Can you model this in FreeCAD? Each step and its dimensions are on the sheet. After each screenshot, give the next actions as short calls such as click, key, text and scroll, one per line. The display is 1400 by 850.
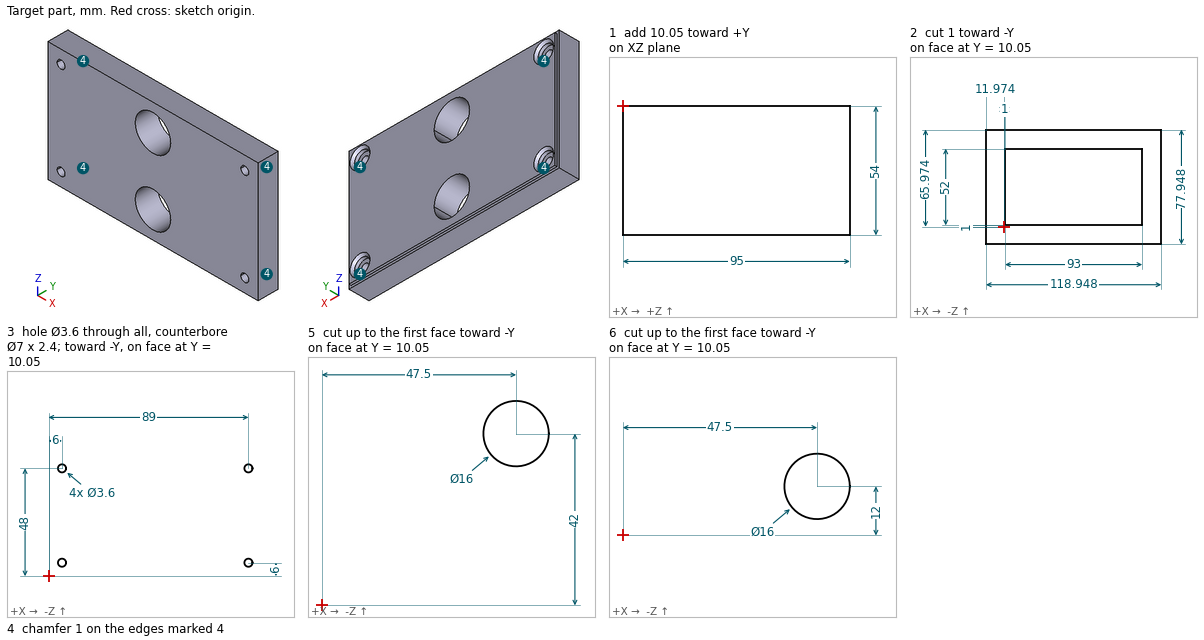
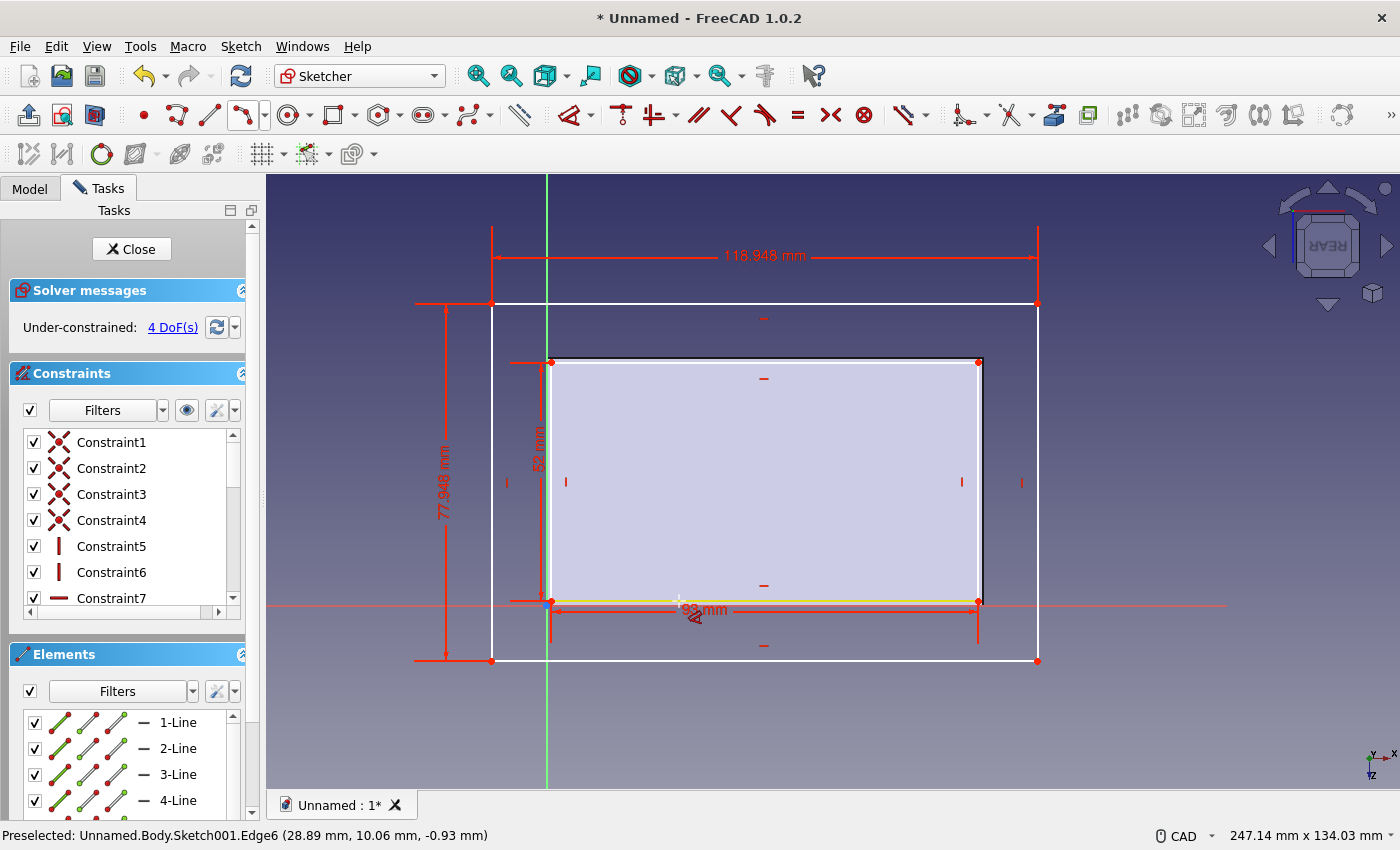
scroll(551, 363, up, 11)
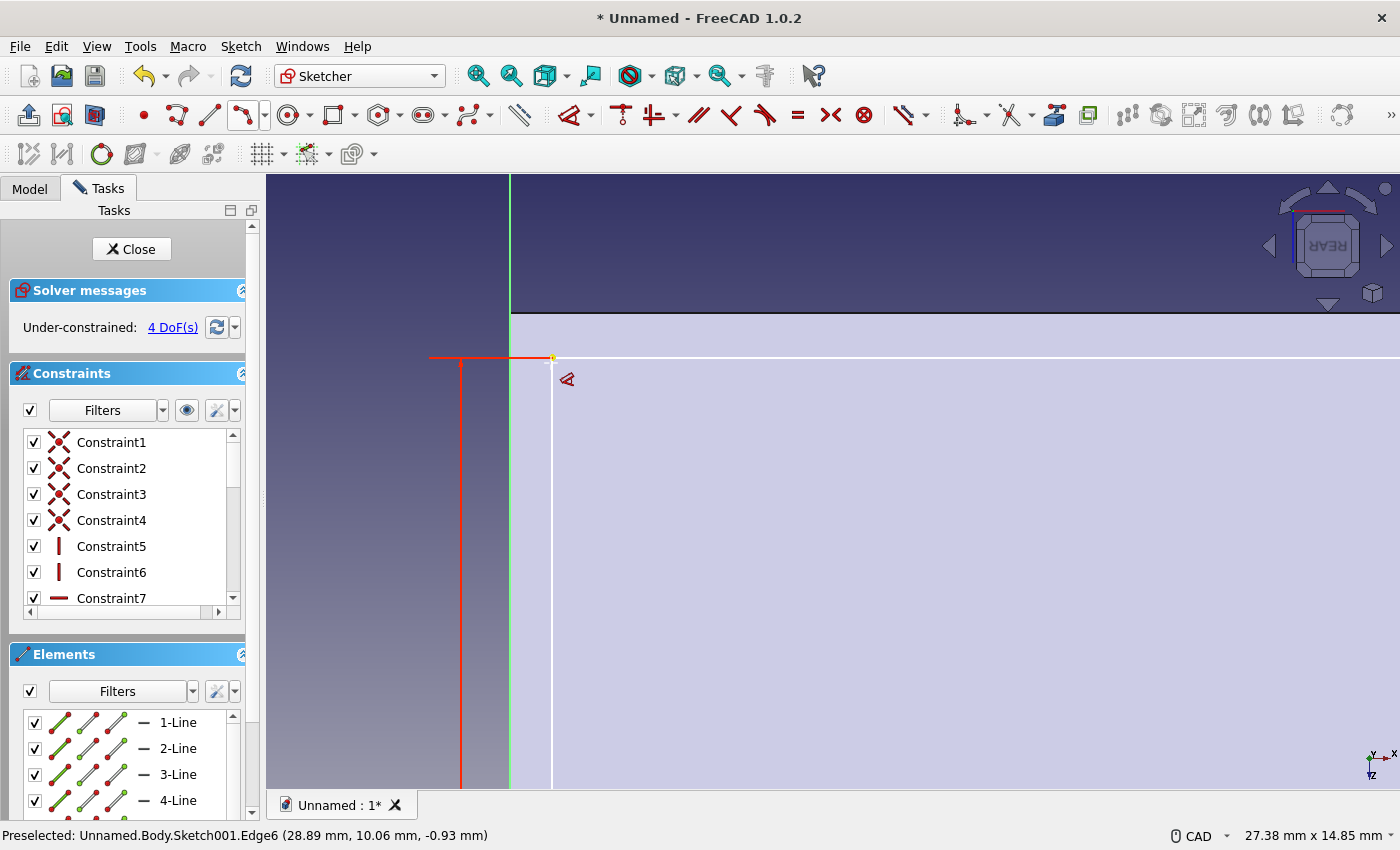
click(552, 358)
click(531, 324)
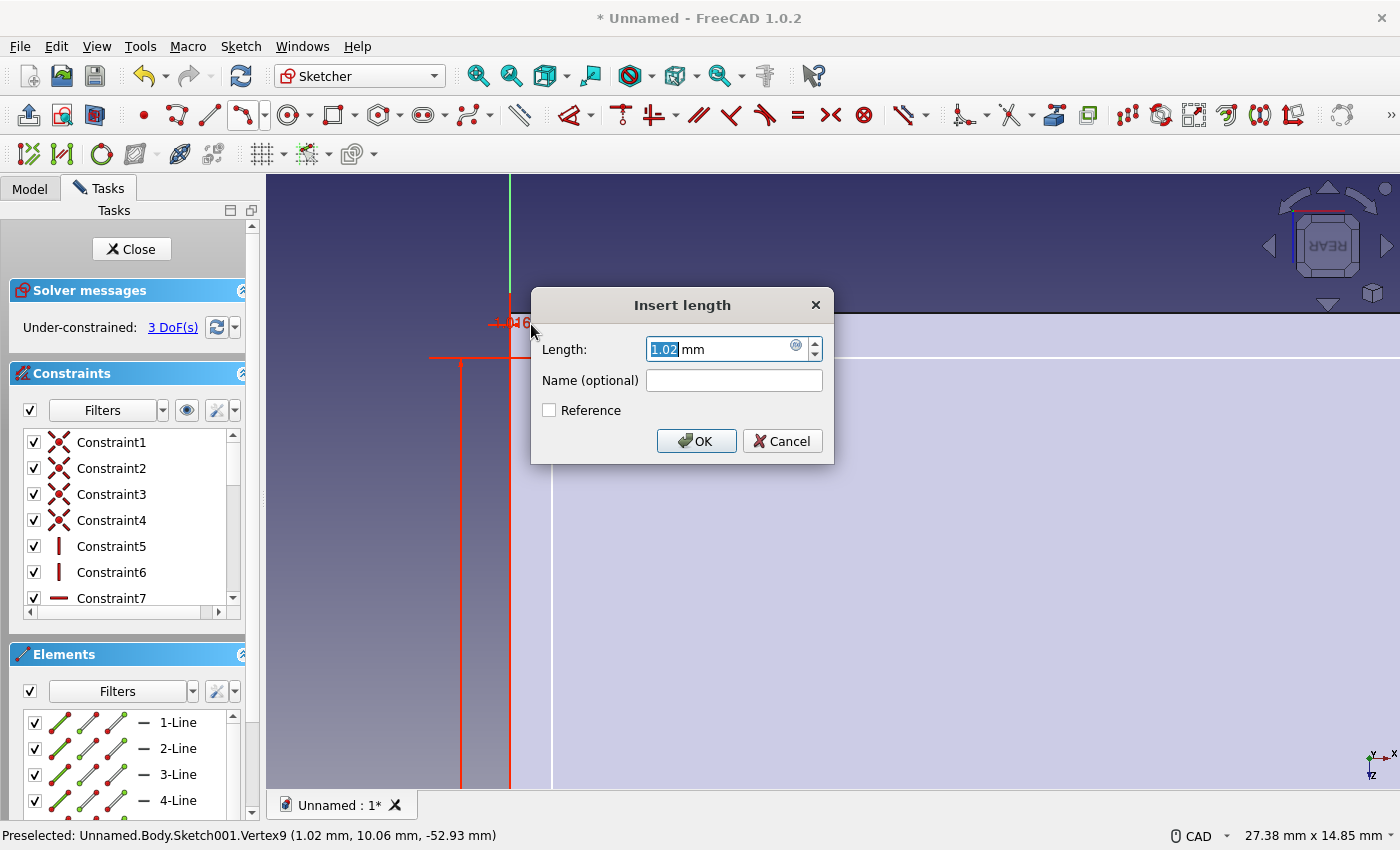
text(1)
key(Return)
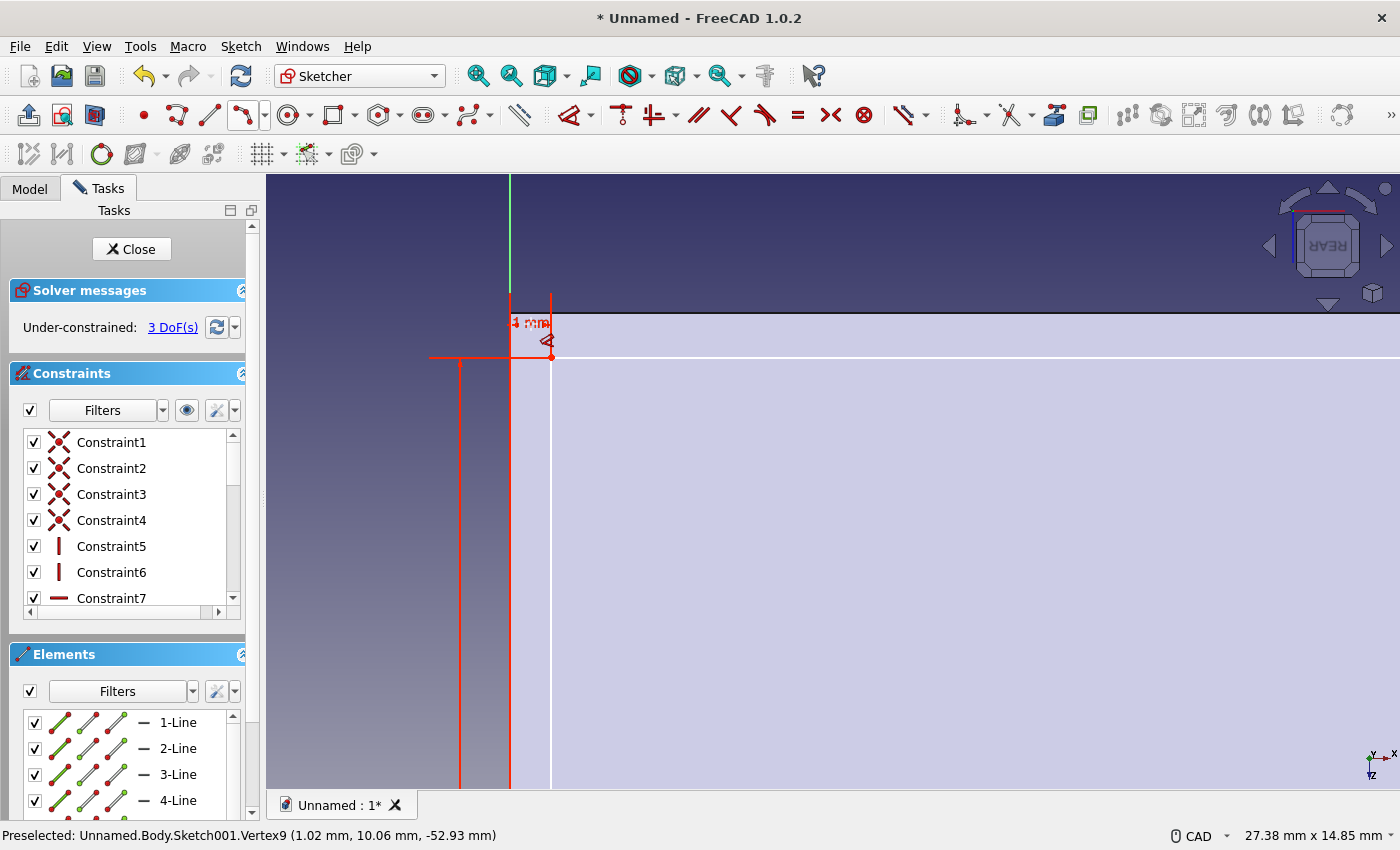
scroll(551, 363, down, 11)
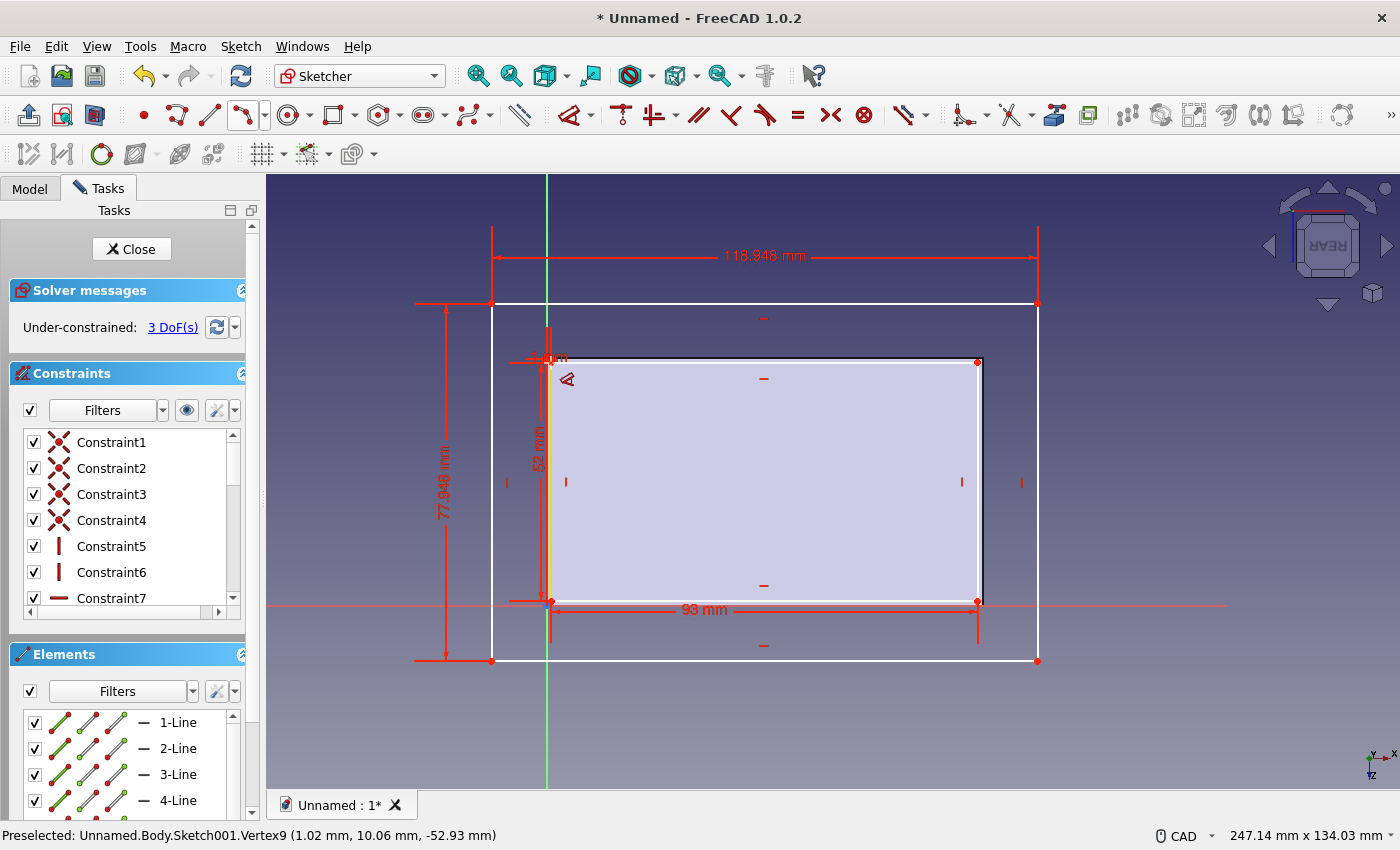
scroll(551, 601, up, 11)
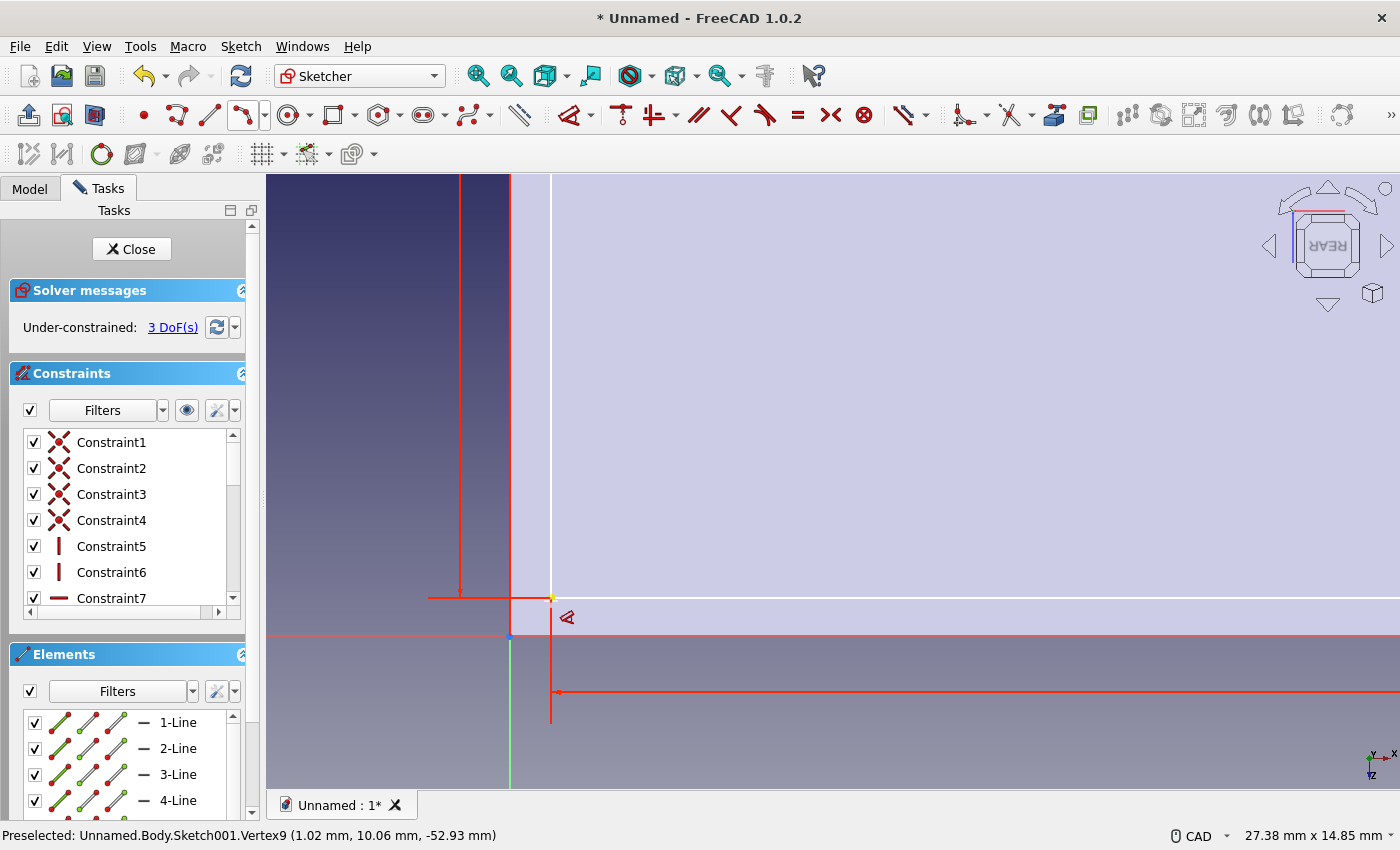
click(551, 598)
click(476, 617)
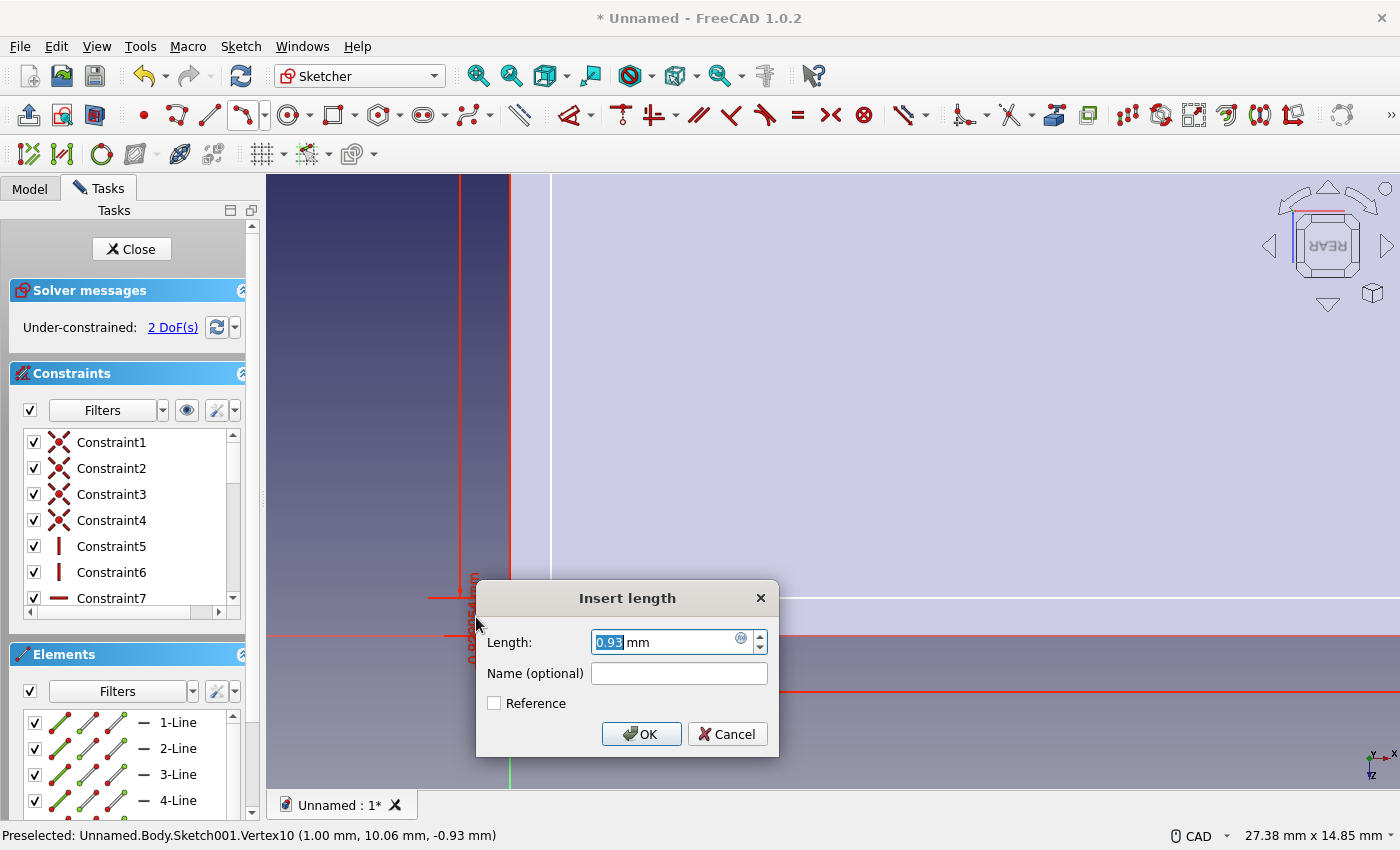
text(1)
key(Return)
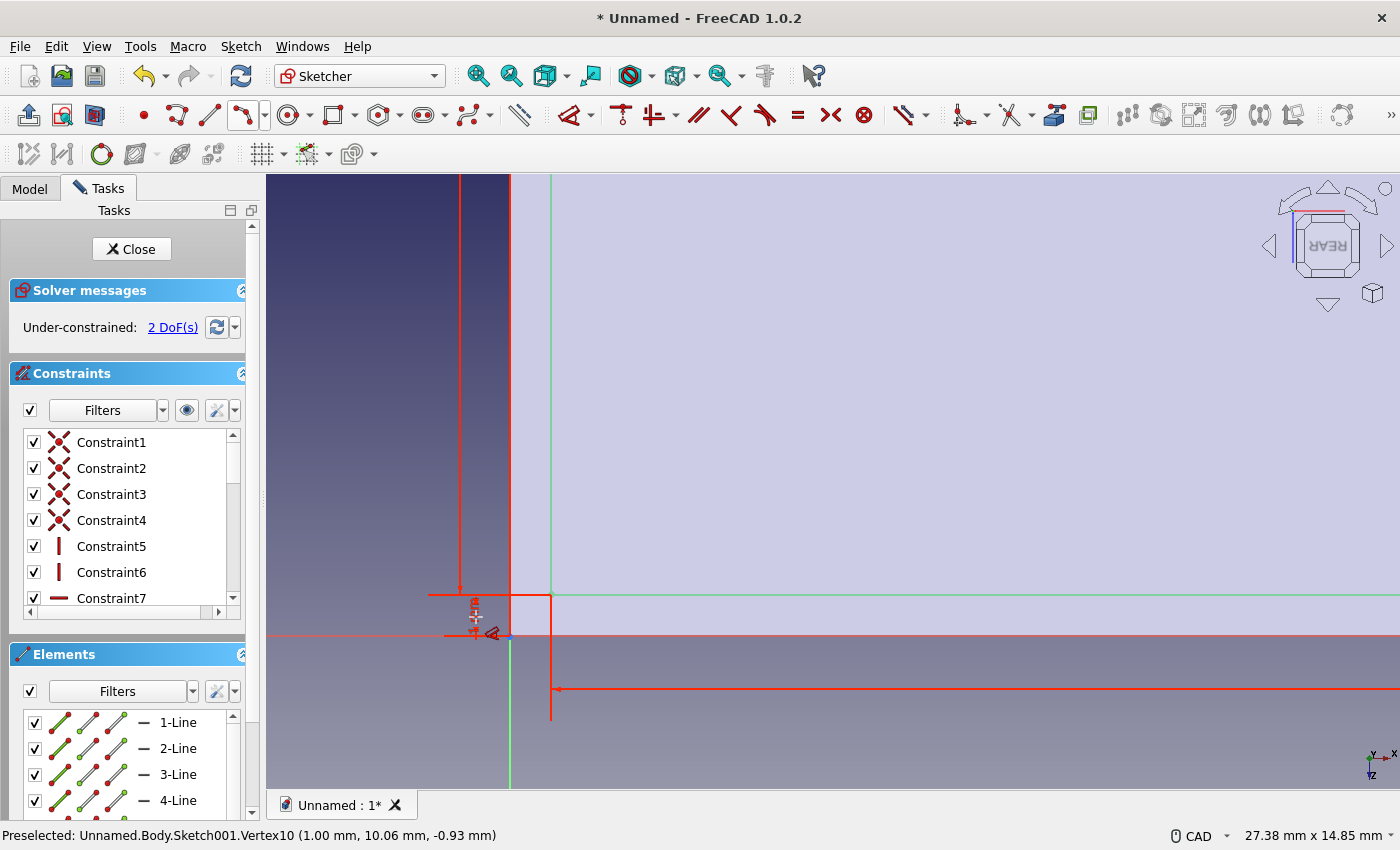
scroll(551, 602, down, 11)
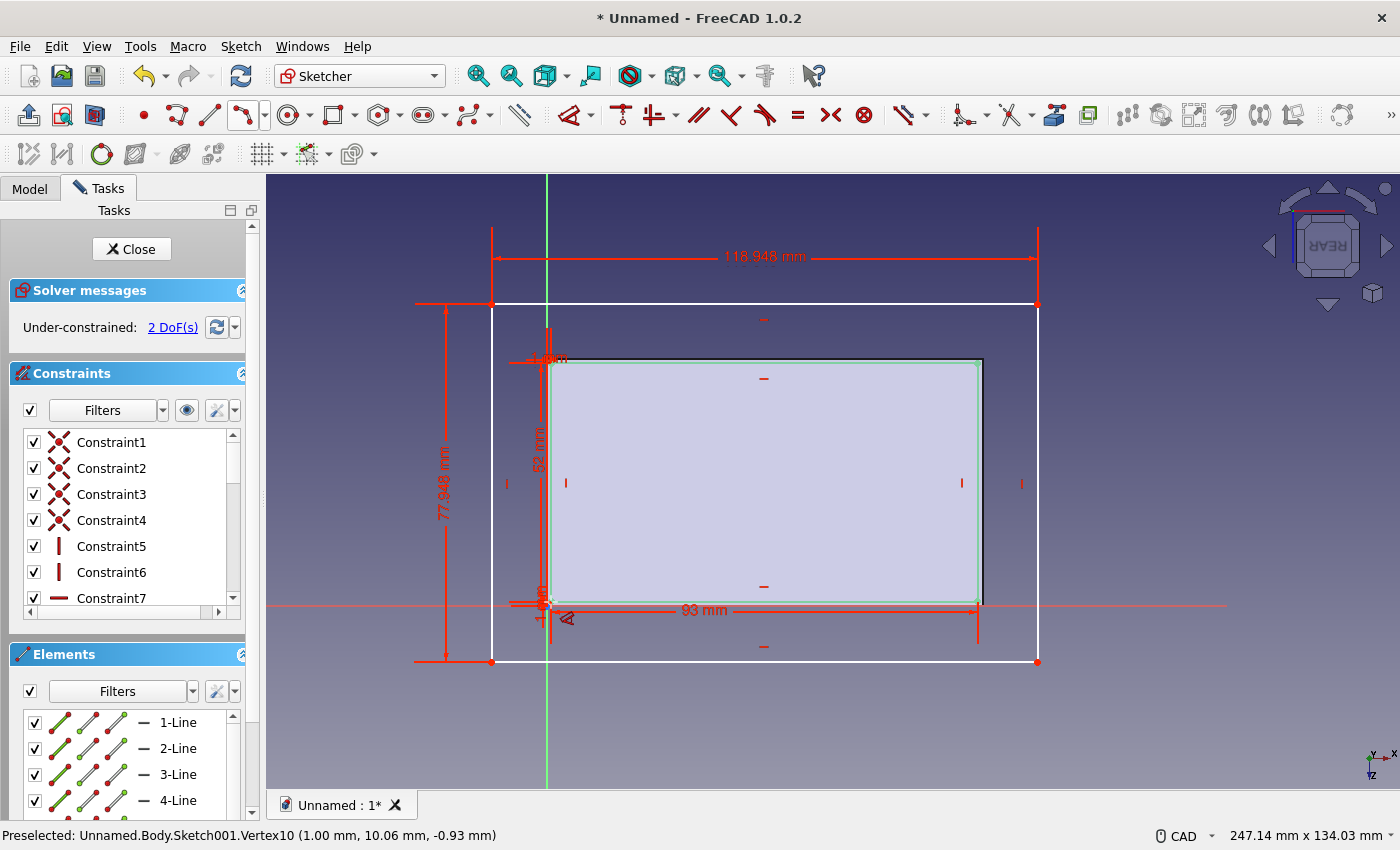
click(492, 304)
click(519, 270)